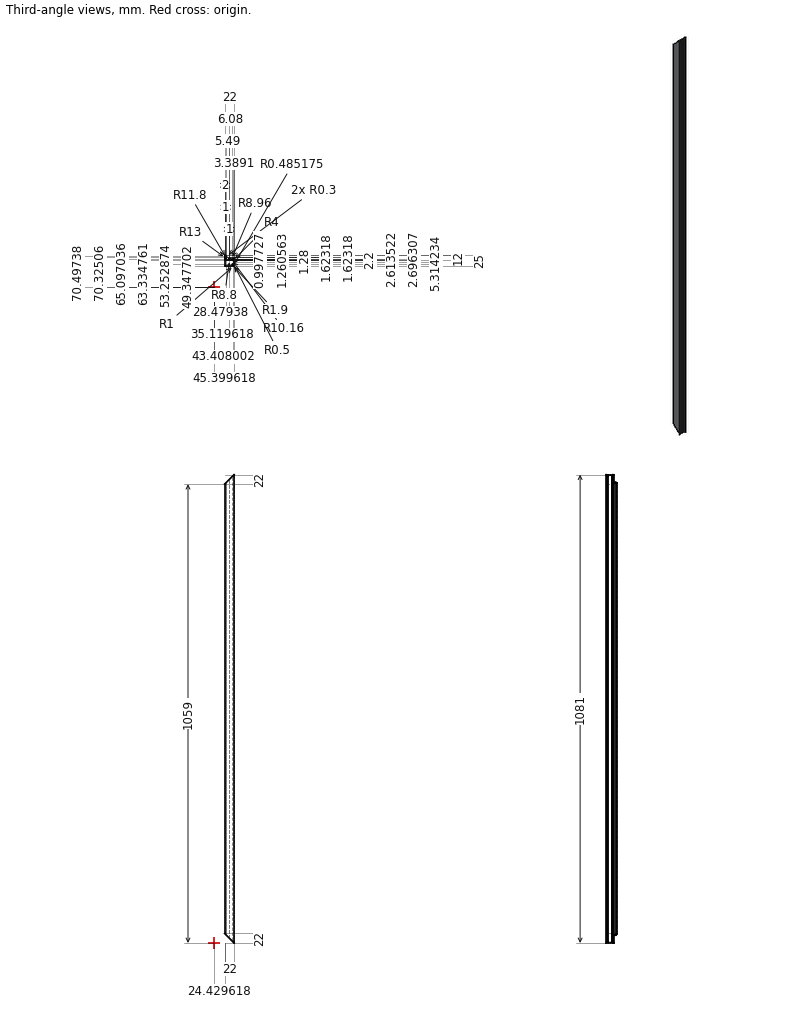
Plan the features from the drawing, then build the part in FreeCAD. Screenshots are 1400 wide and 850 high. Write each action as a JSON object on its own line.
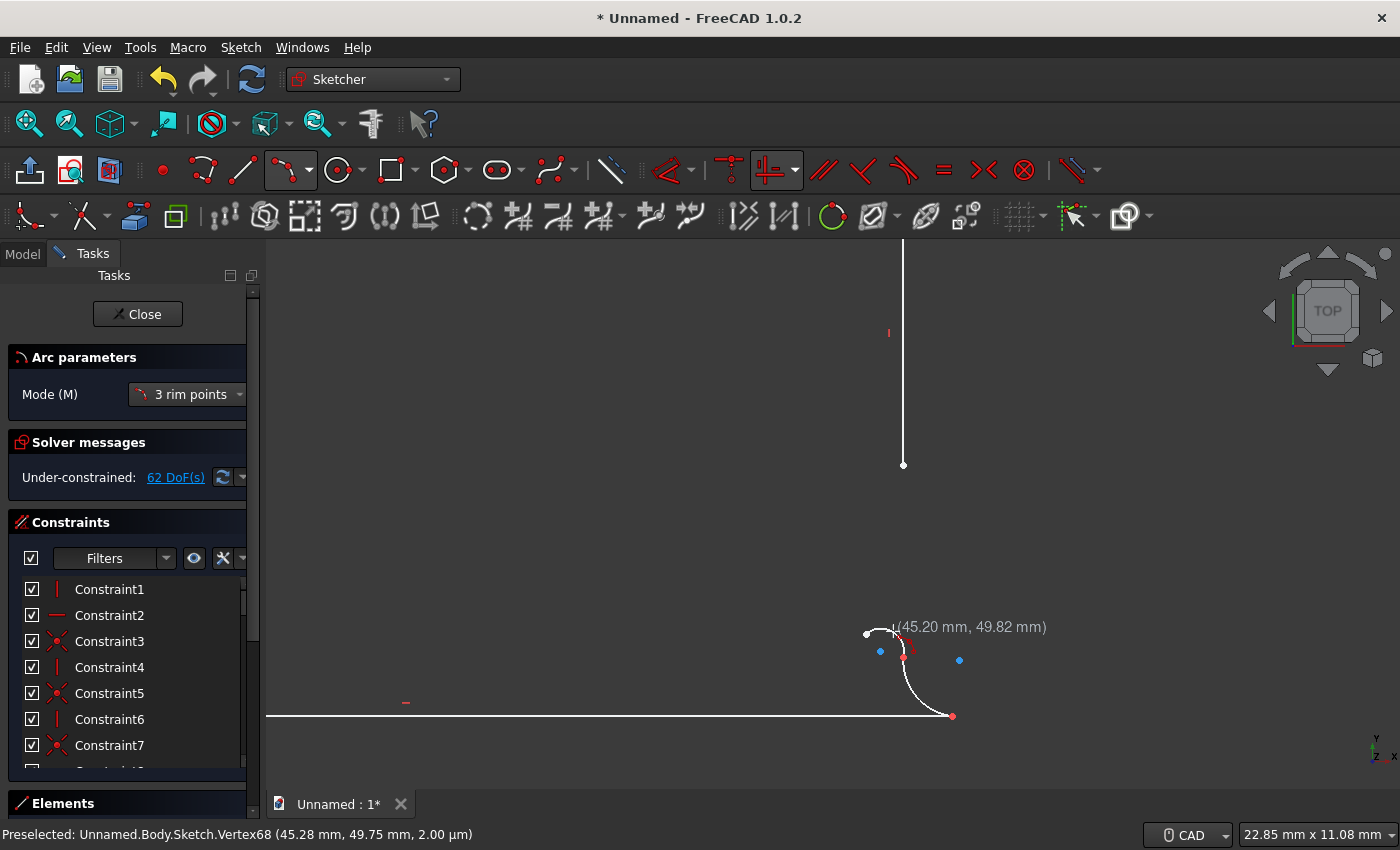
{"action": "left_click", "coordinate": [866, 634]}
{"action": "left_click", "coordinate": [864, 482]}
{"action": "left_click", "coordinate": [714, 560]}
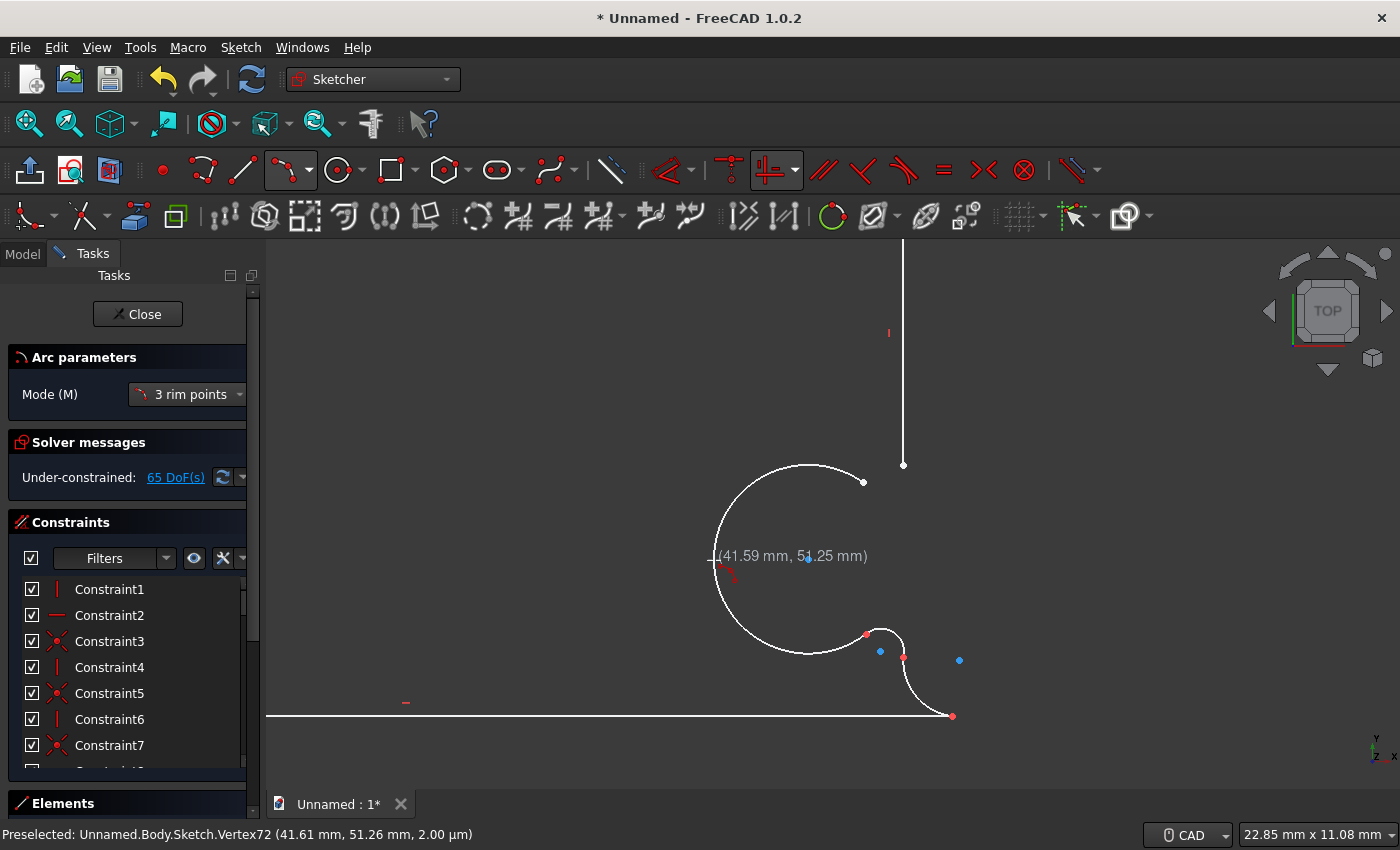
{"action": "left_click", "coordinate": [864, 483]}
{"action": "left_click", "coordinate": [903, 465]}
{"action": "left_click", "coordinate": [889, 484]}
{"action": "key", "text": "Escape"}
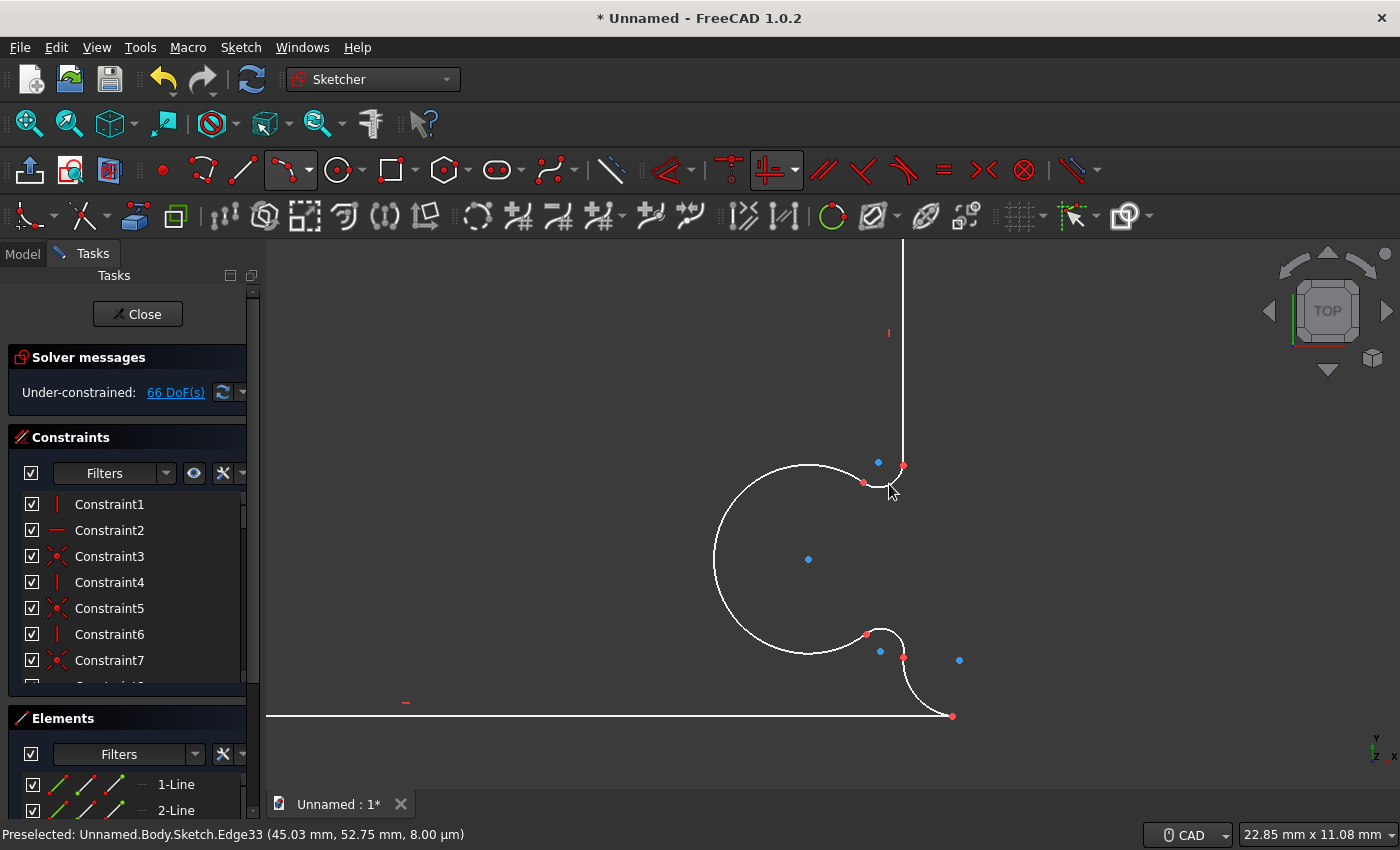
{"action": "left_click", "coordinate": [903, 385]}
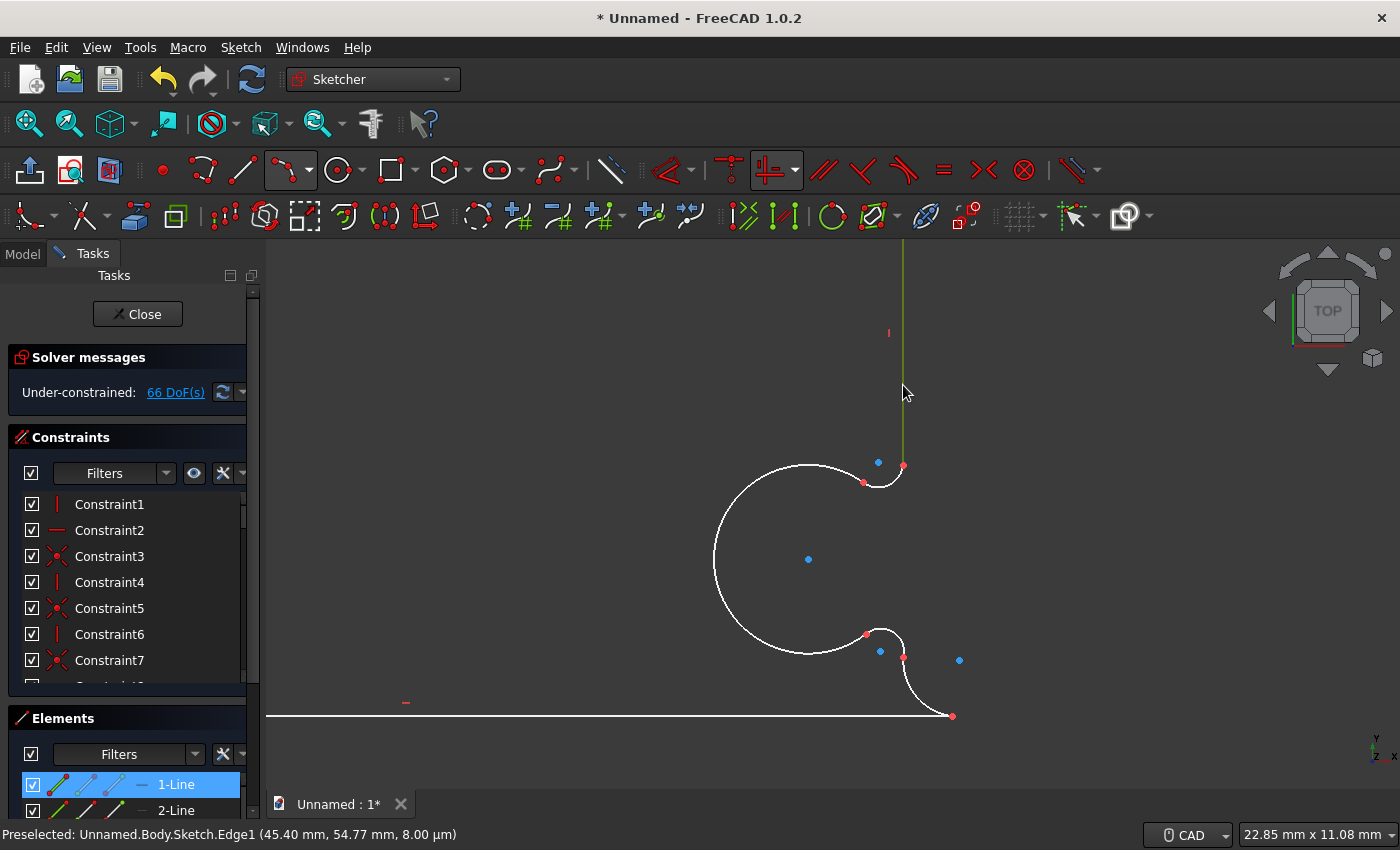
{"action": "scroll", "coordinate": [918, 696], "scroll_direction": "down", "scroll_amount": 6}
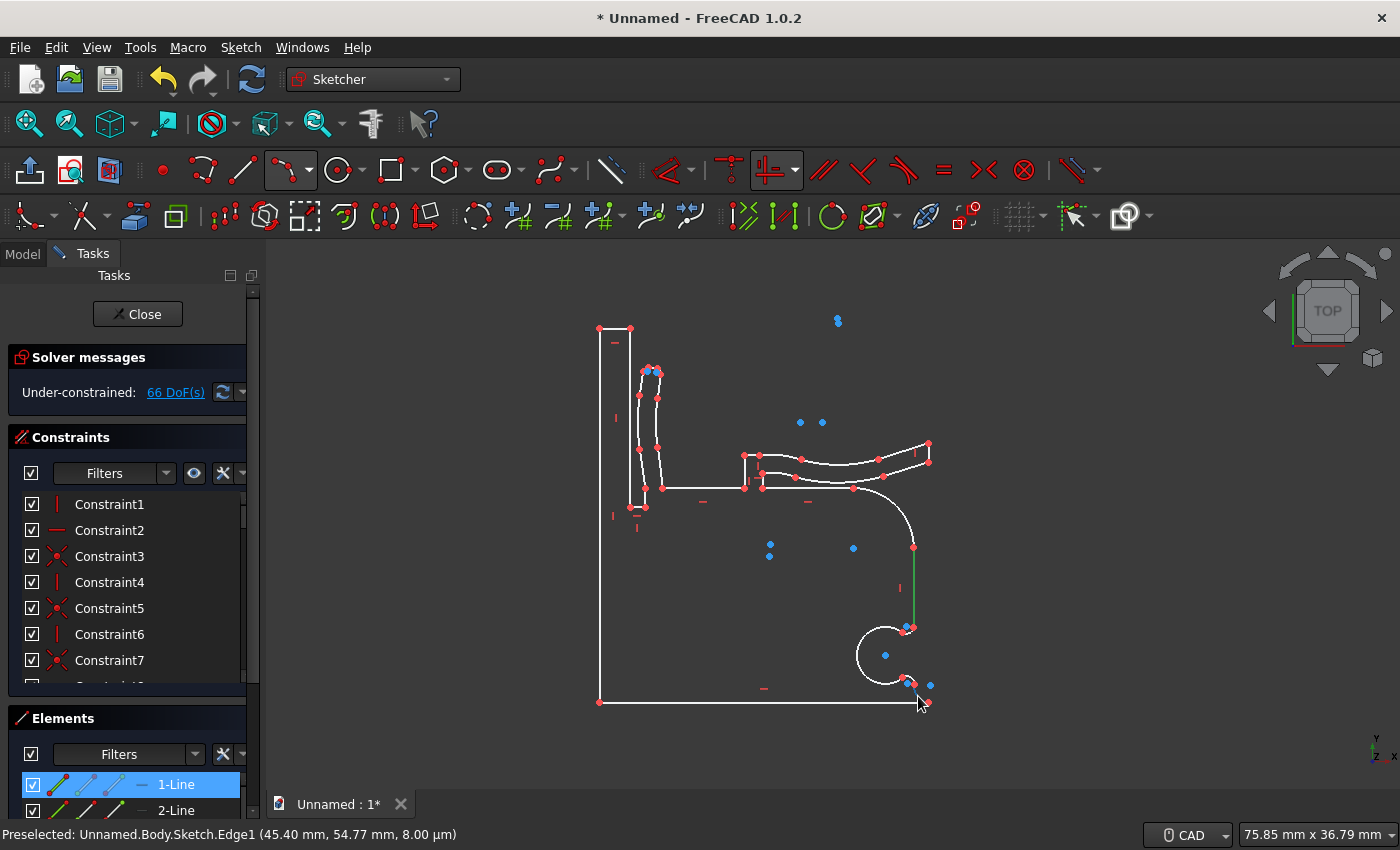
{"action": "left_click", "coordinate": [907, 520]}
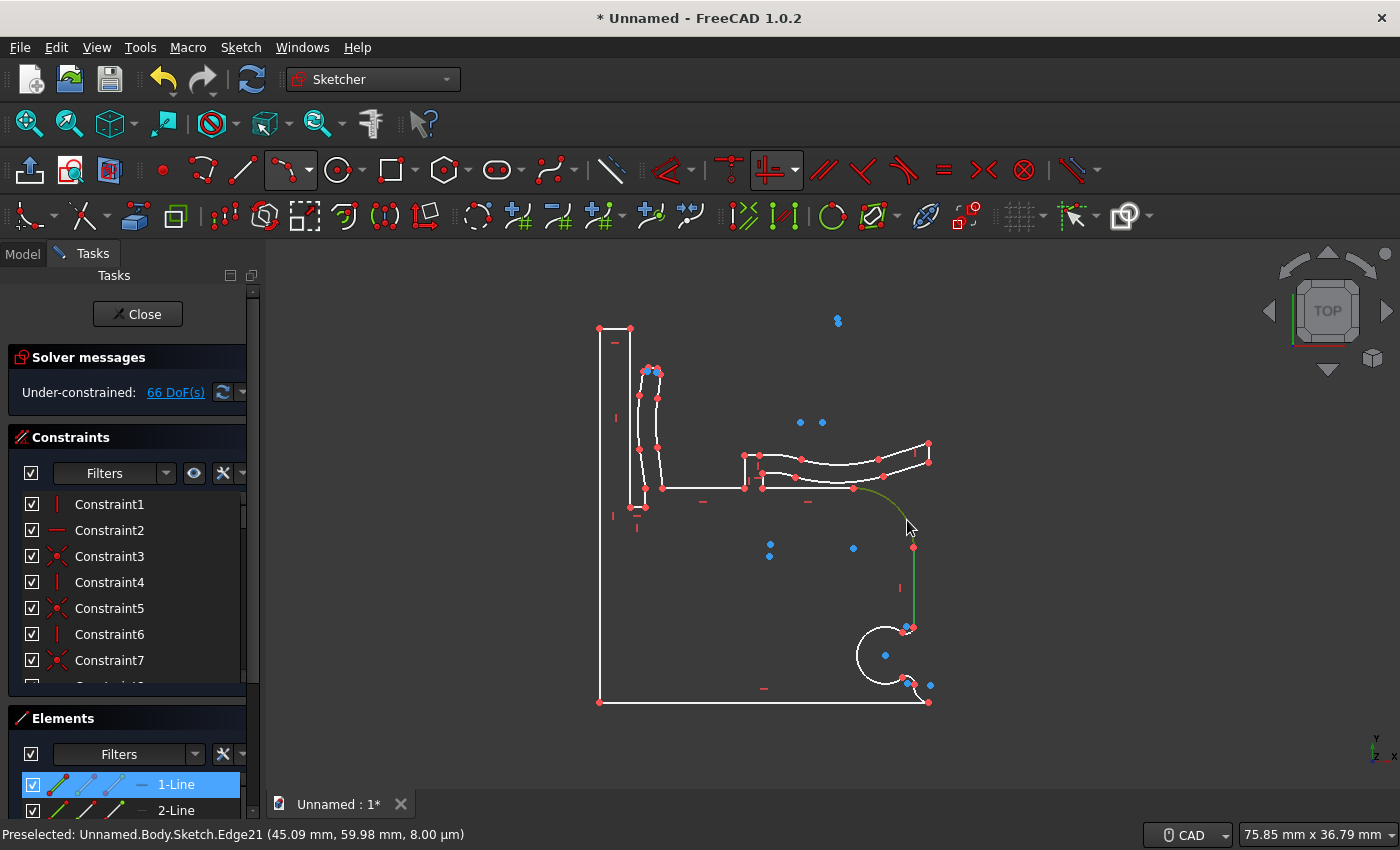
{"action": "left_click", "coordinate": [904, 170]}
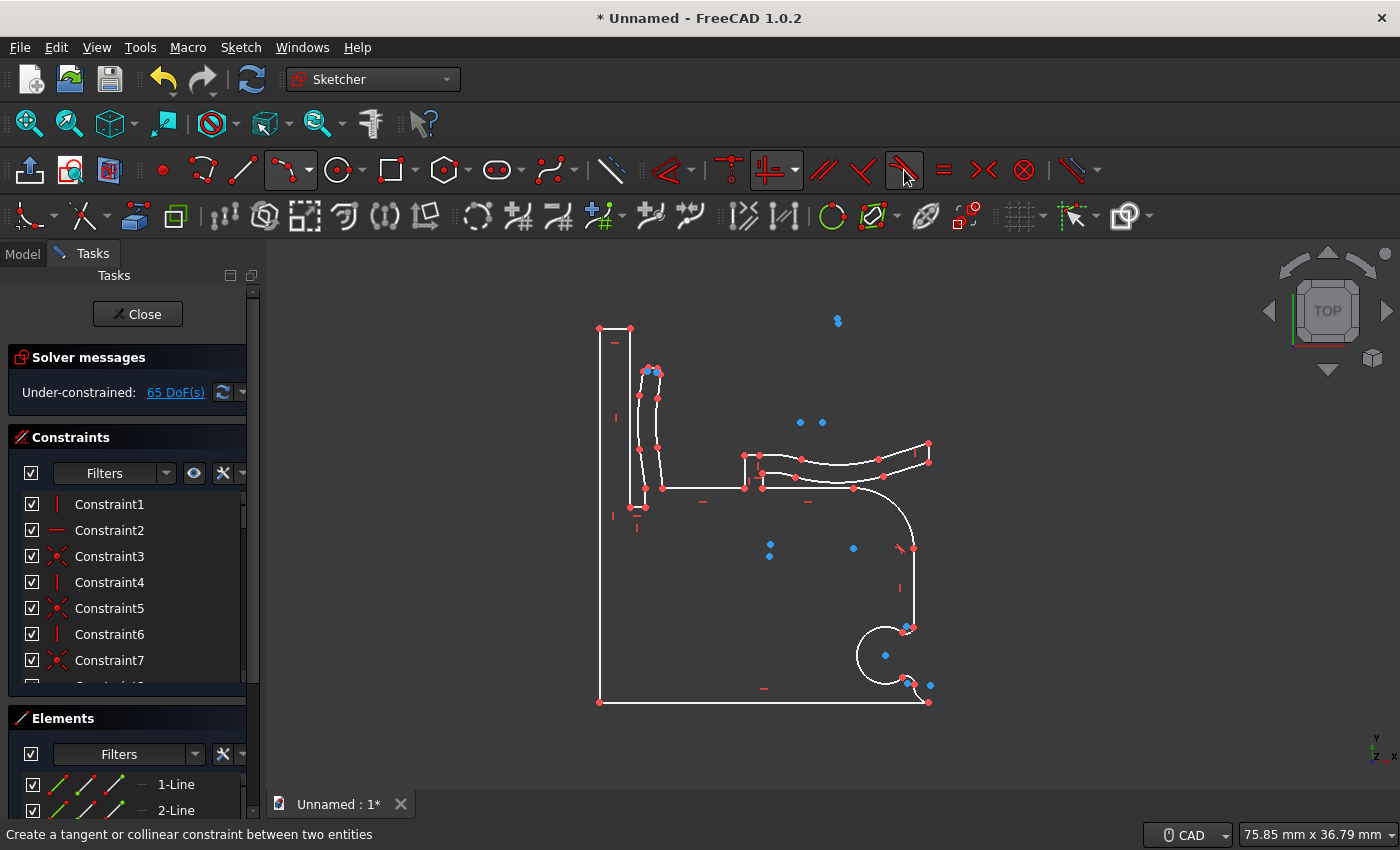
{"action": "left_click", "coordinate": [914, 604]}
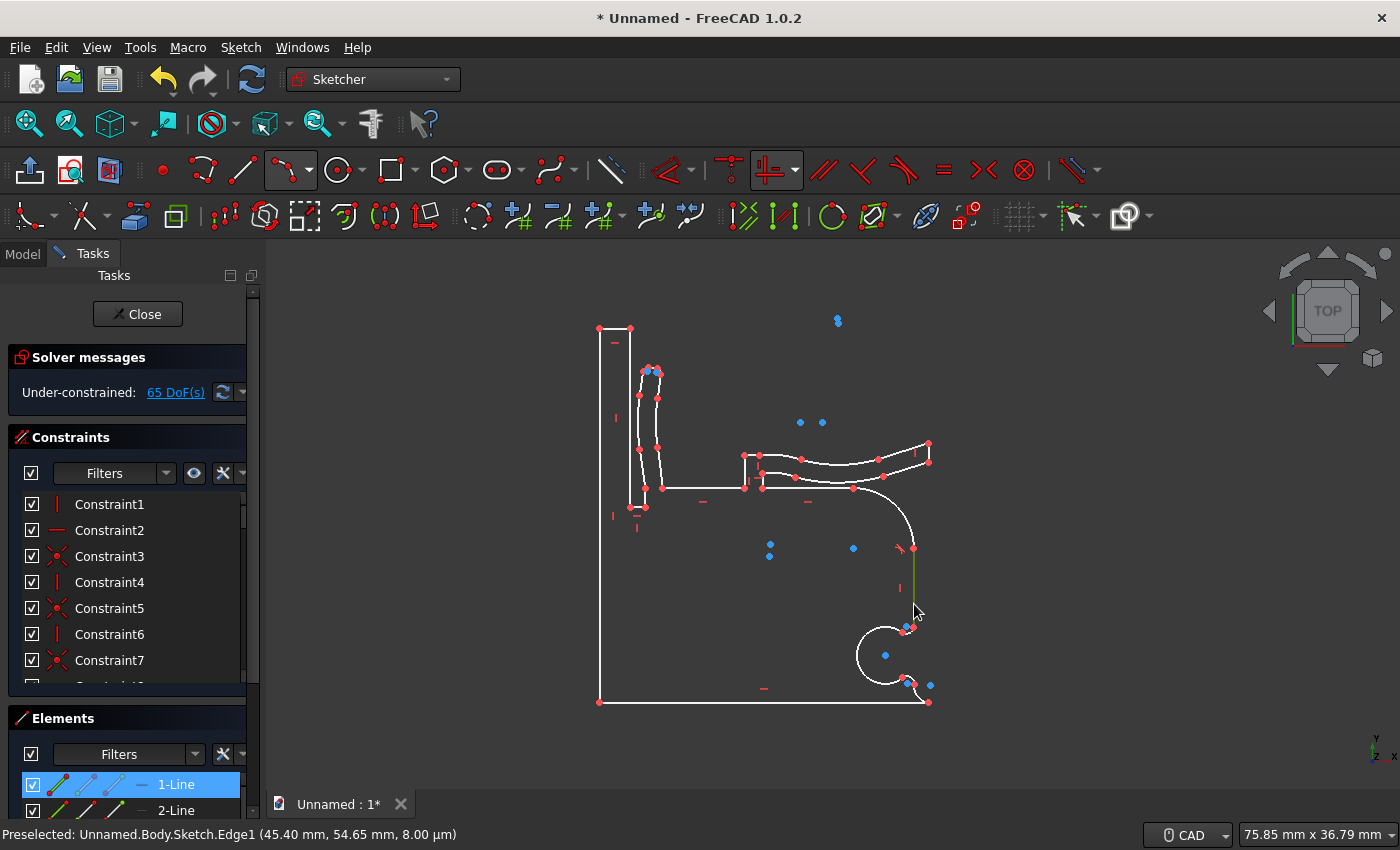
{"action": "scroll", "coordinate": [910, 633], "scroll_direction": "up", "scroll_amount": 4}